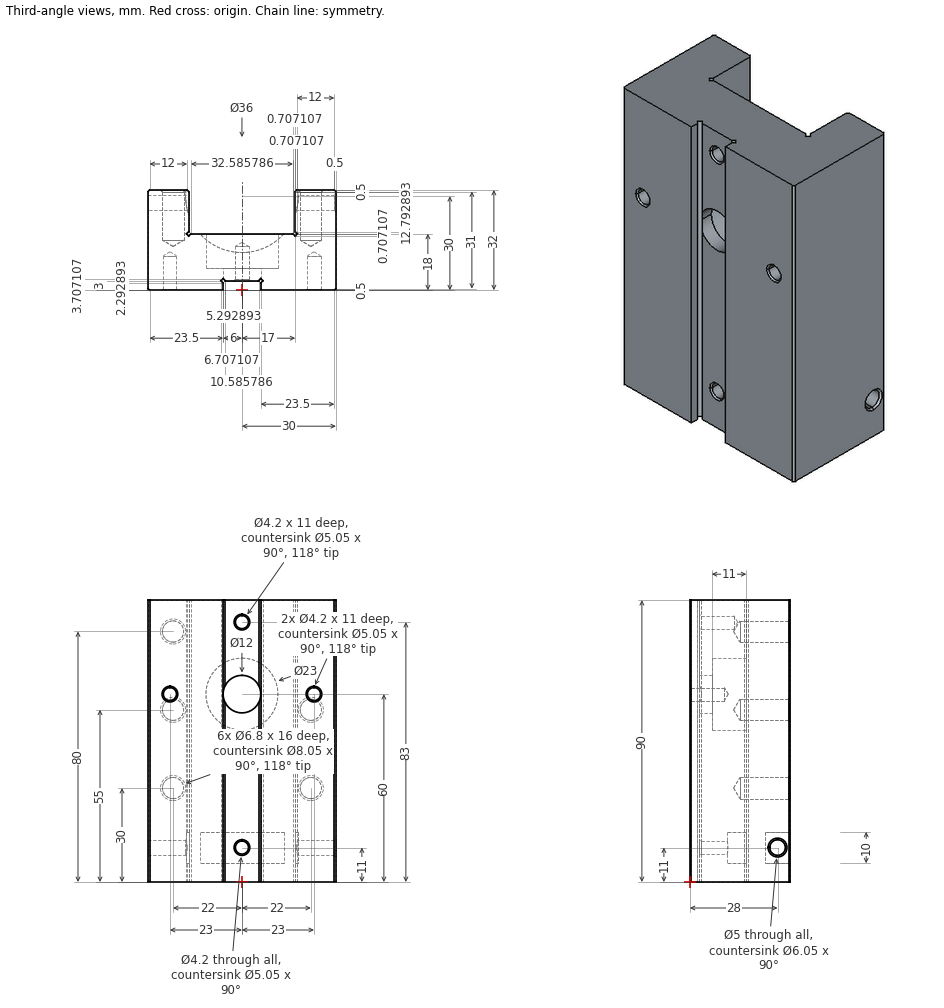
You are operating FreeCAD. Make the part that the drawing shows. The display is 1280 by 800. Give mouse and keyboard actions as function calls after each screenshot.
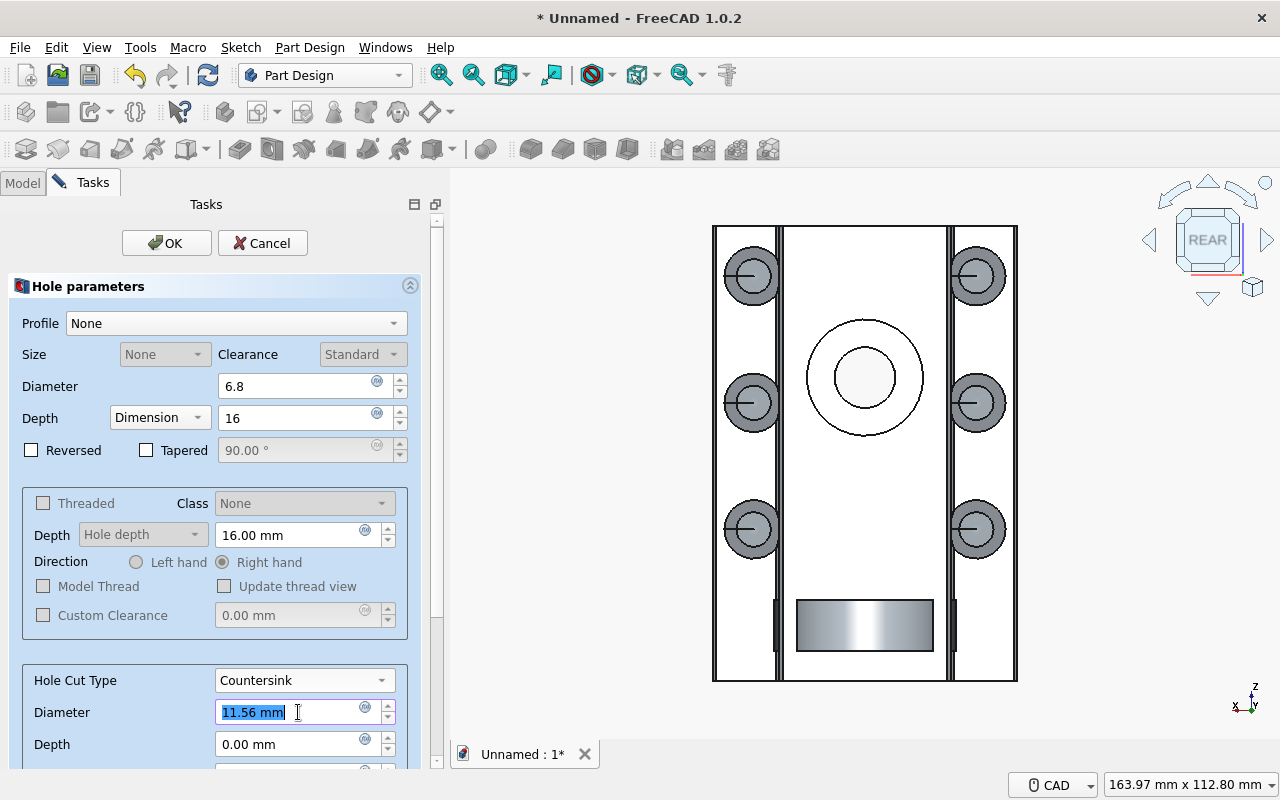
text(8.05)
key(Tab)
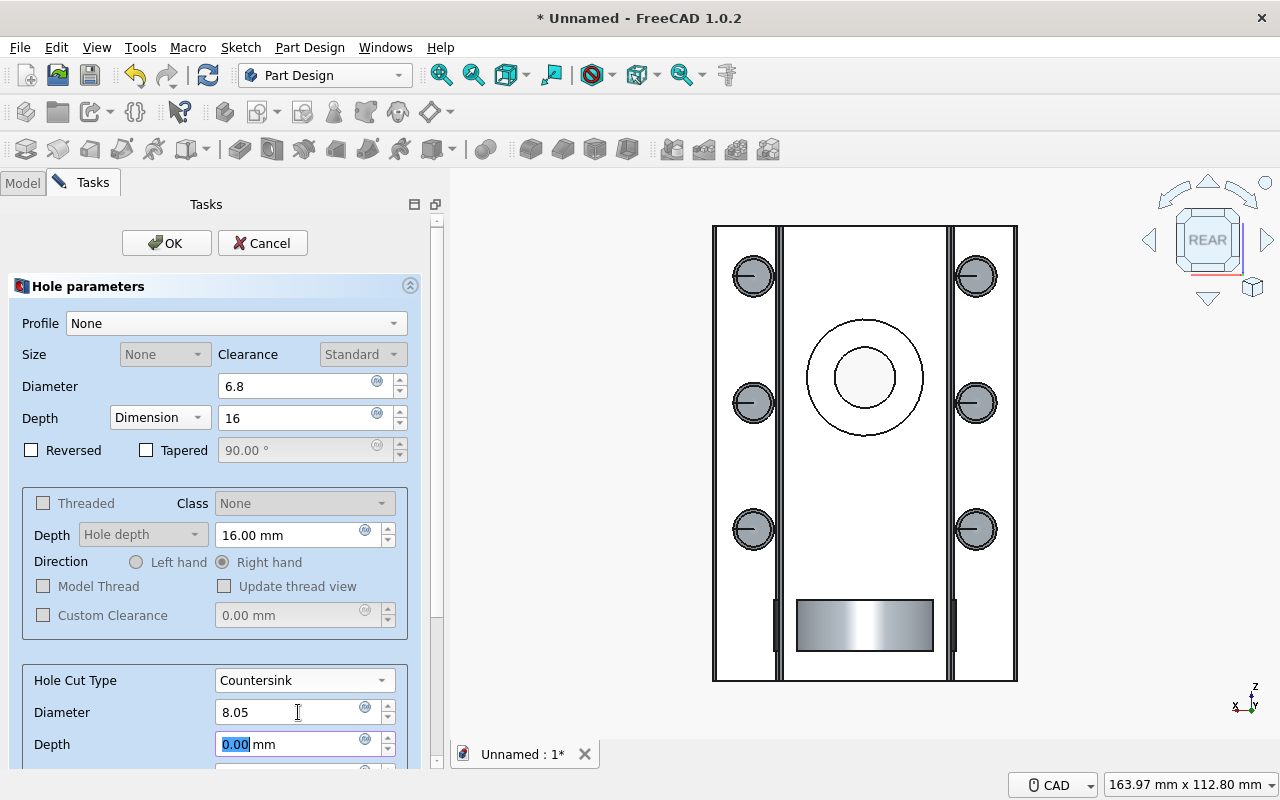
click(167, 243)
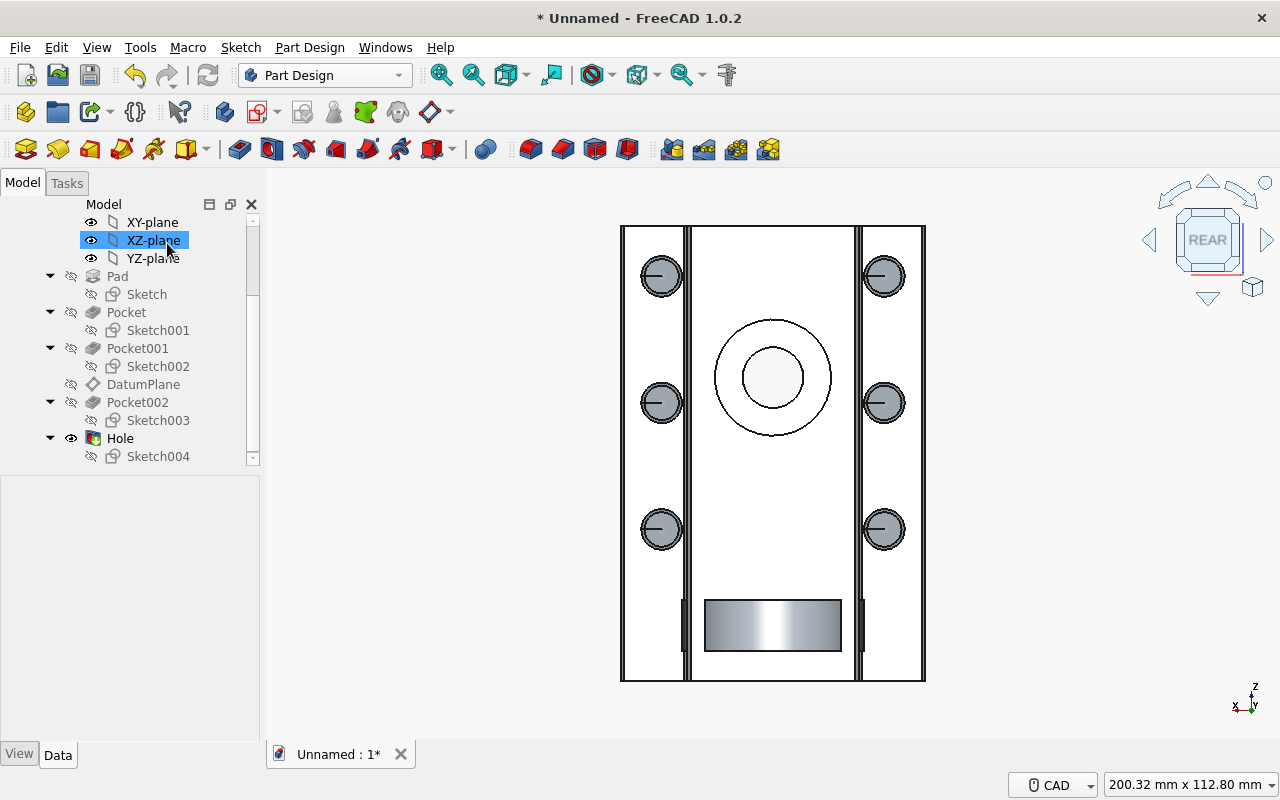
key(0)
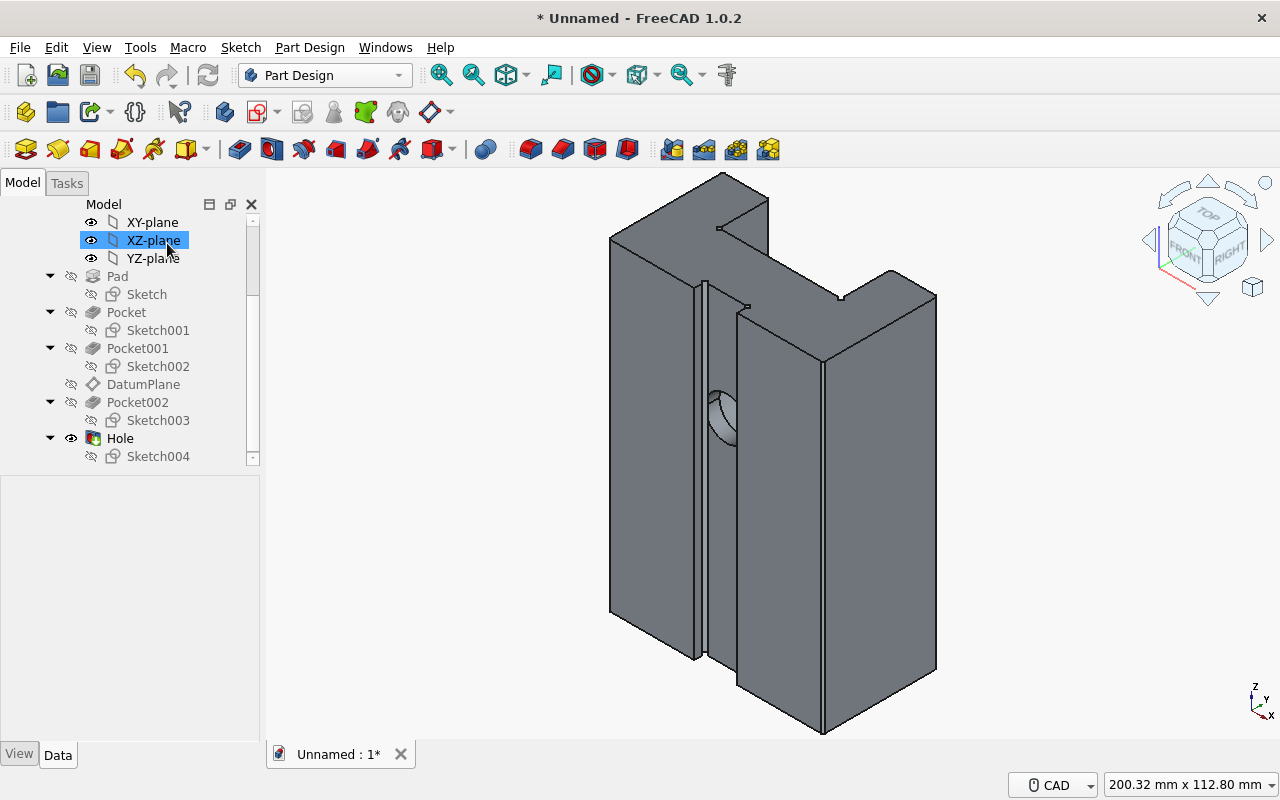
click(880, 408)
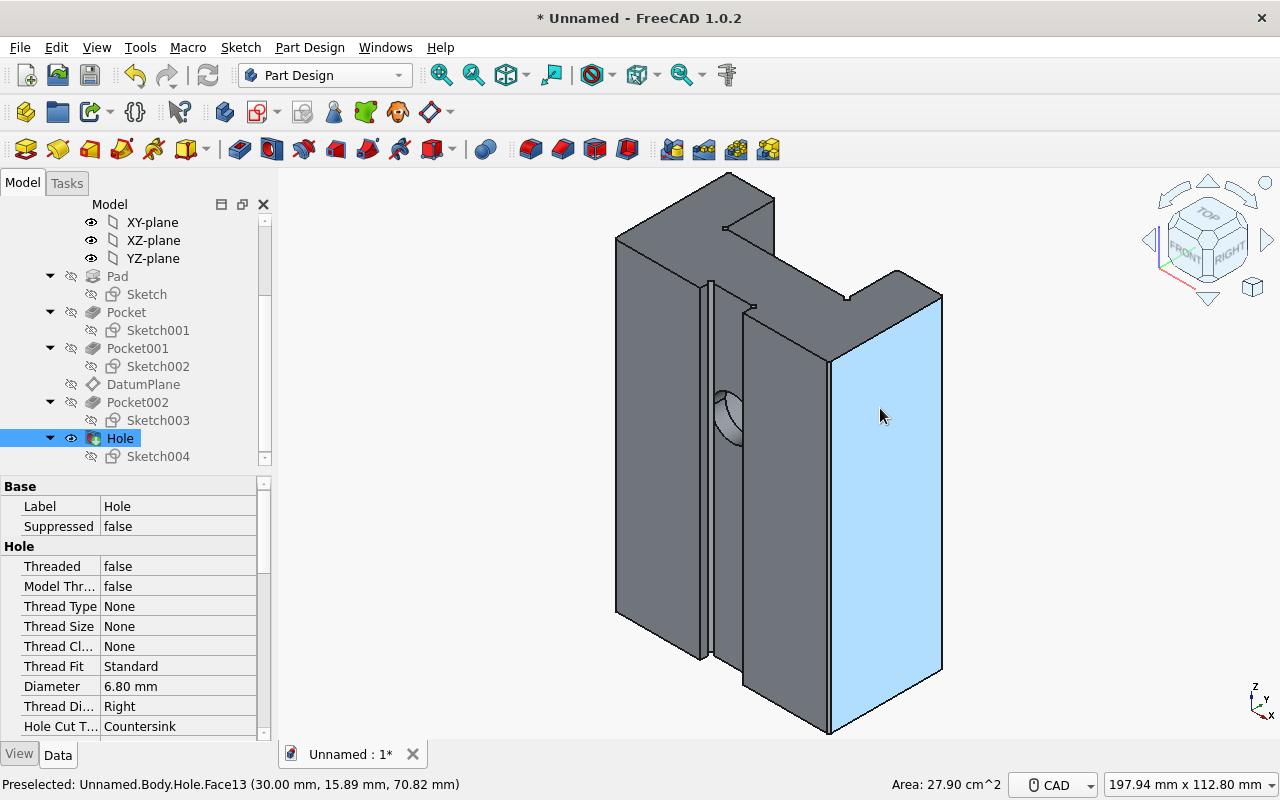
click(258, 112)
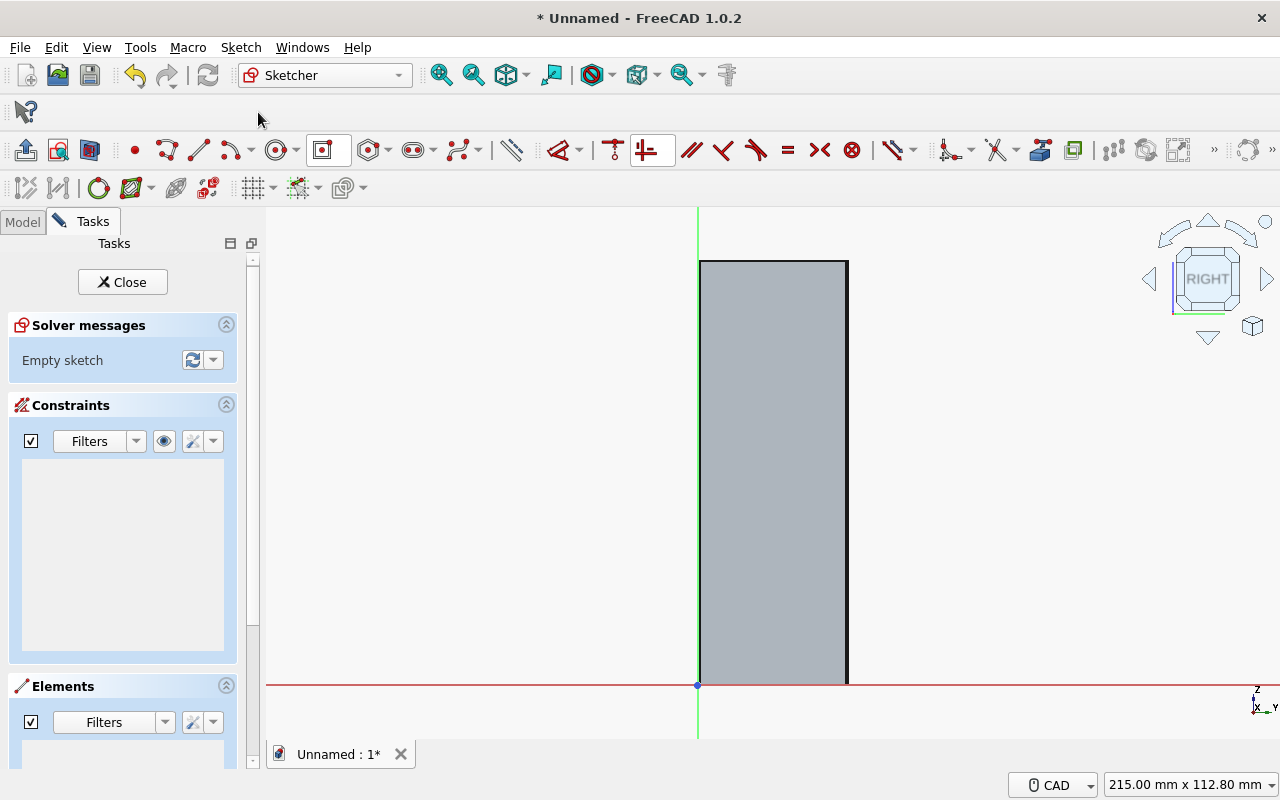
scroll(840, 646, up, 13)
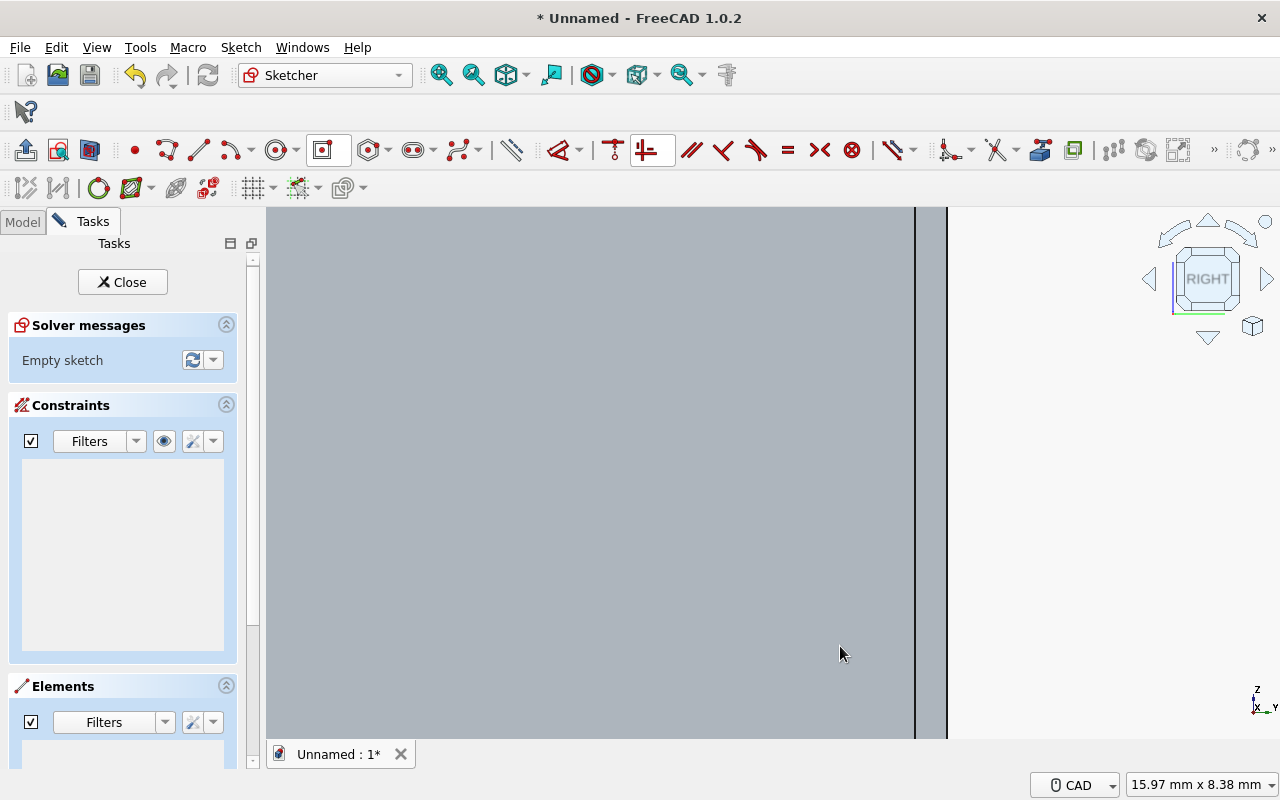
click(276, 150)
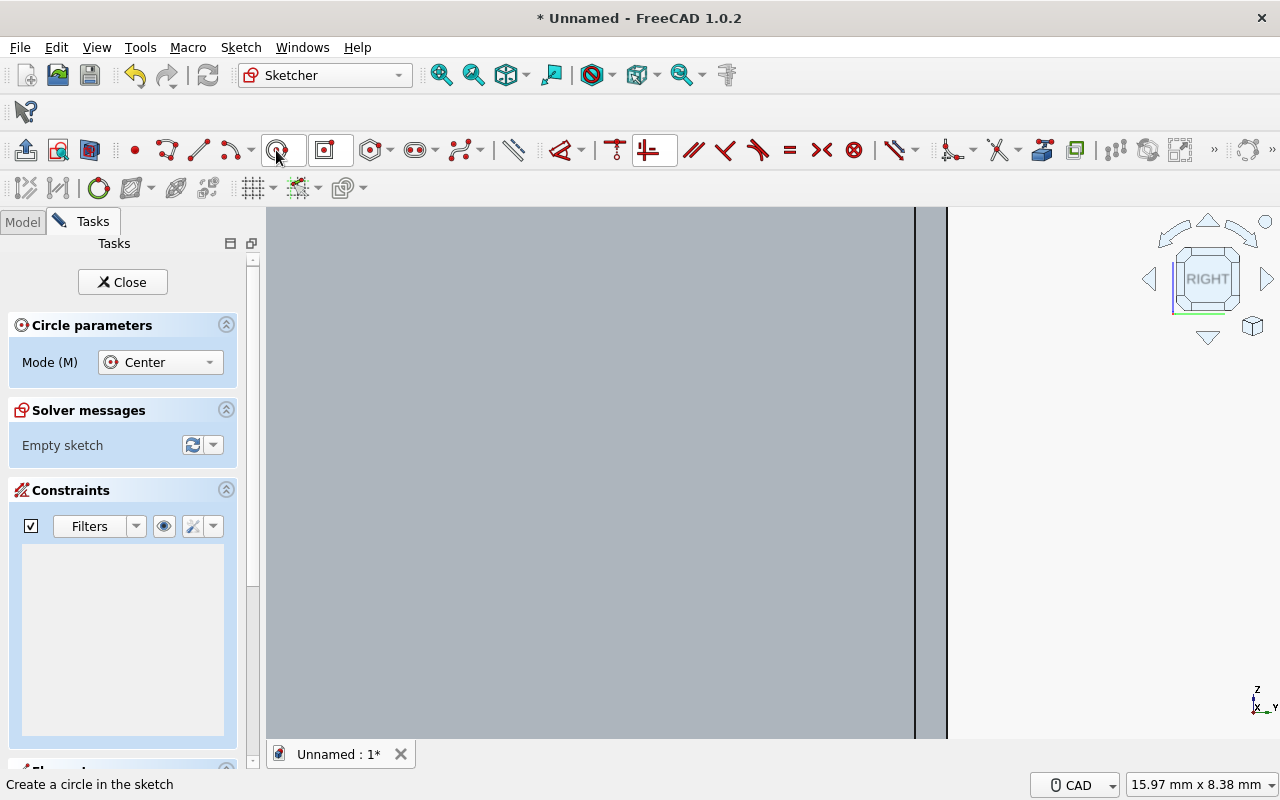
click(693, 465)
move(805, 353)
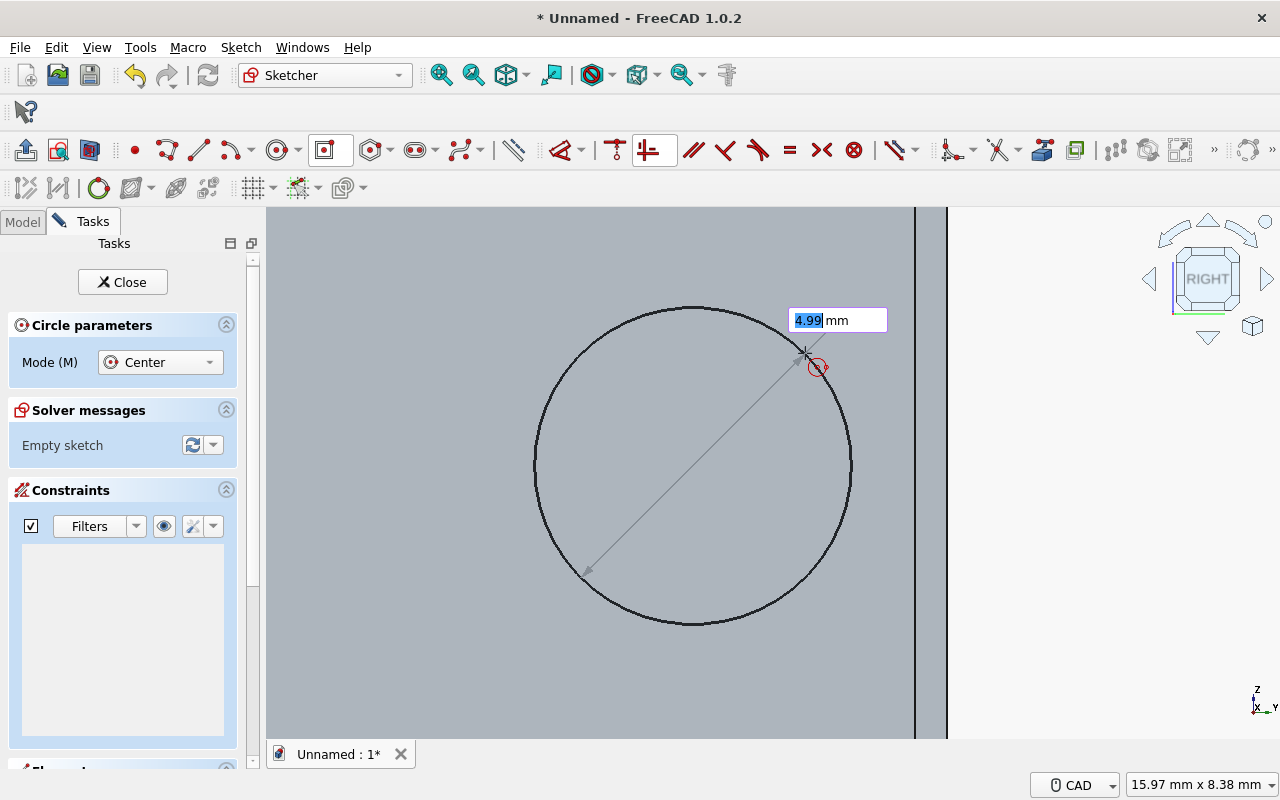
text(5)
key(Return)
key(Escape)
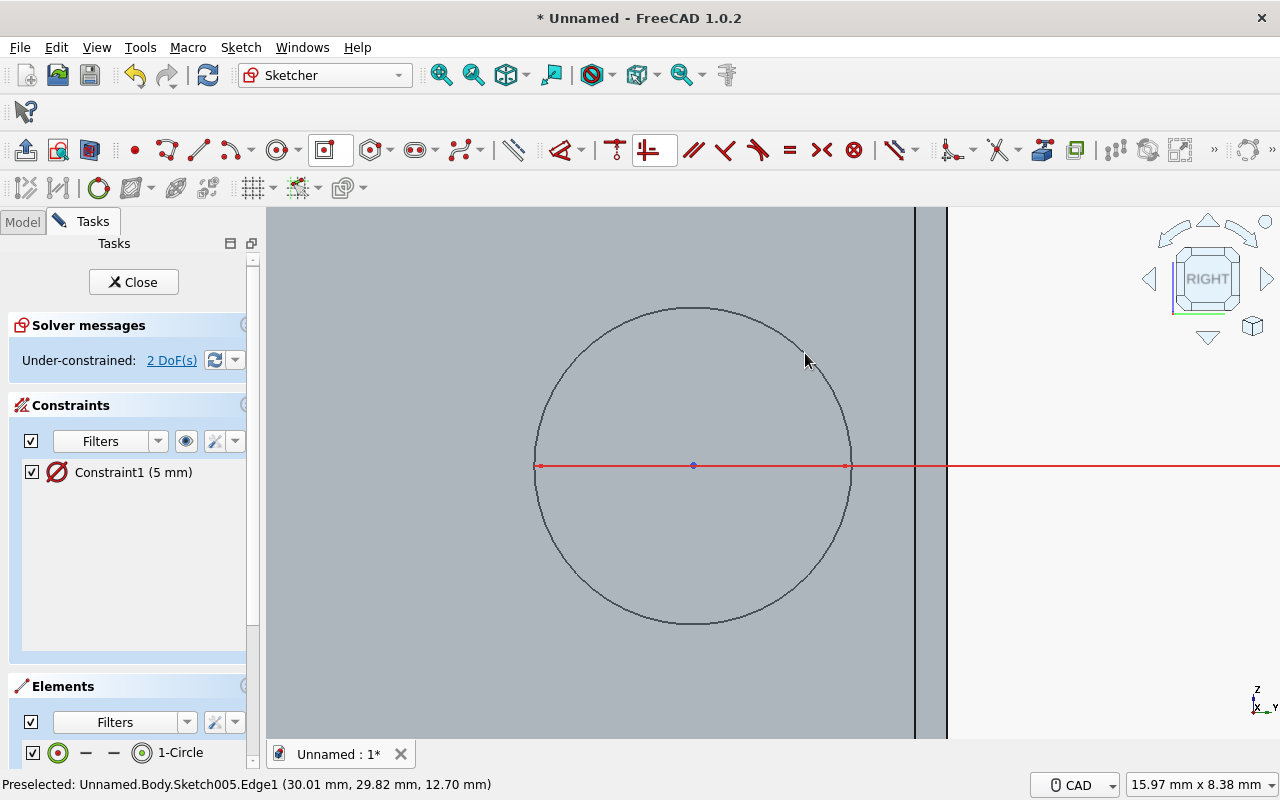
click(560, 150)